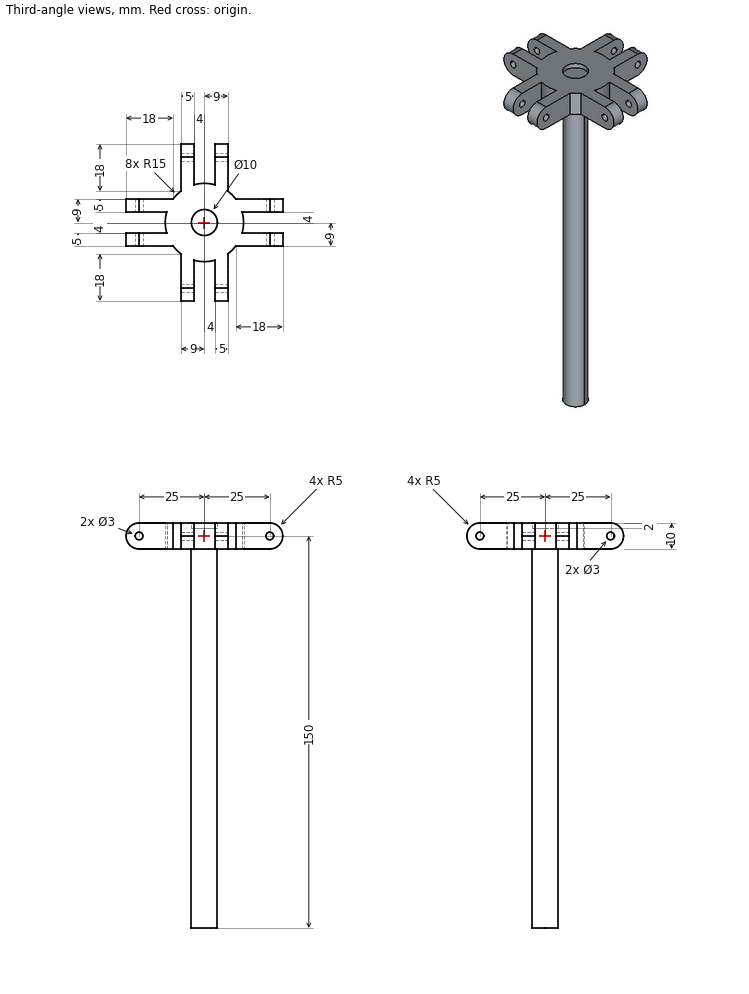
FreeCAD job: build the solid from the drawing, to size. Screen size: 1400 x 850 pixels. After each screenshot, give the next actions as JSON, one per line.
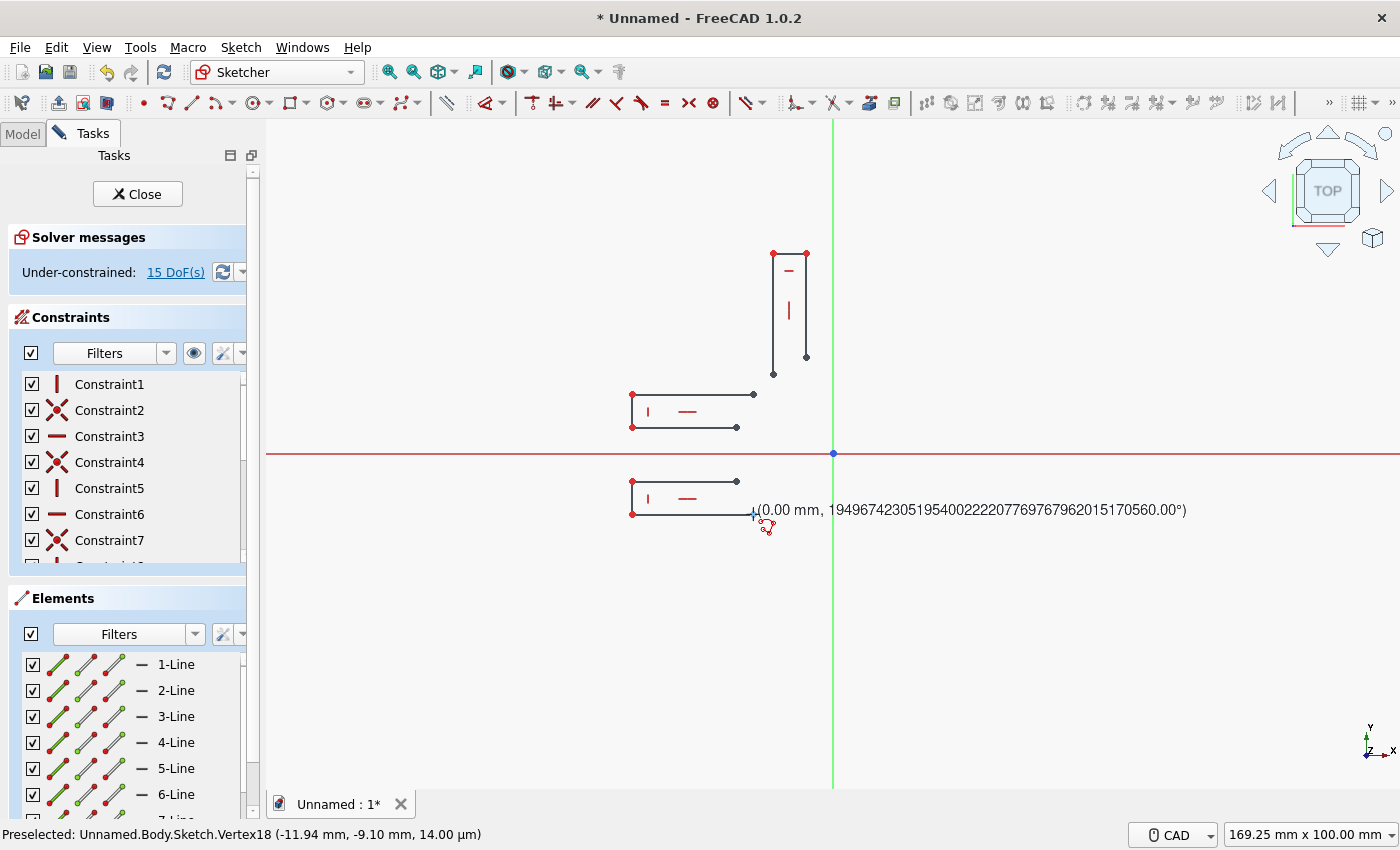
{"action": "left_click", "coordinate": [773, 534]}
{"action": "left_click", "coordinate": [773, 655]}
{"action": "left_click", "coordinate": [806, 655]}
{"action": "left_click", "coordinate": [806, 551]}
{"action": "right_click", "coordinate": [806, 551]}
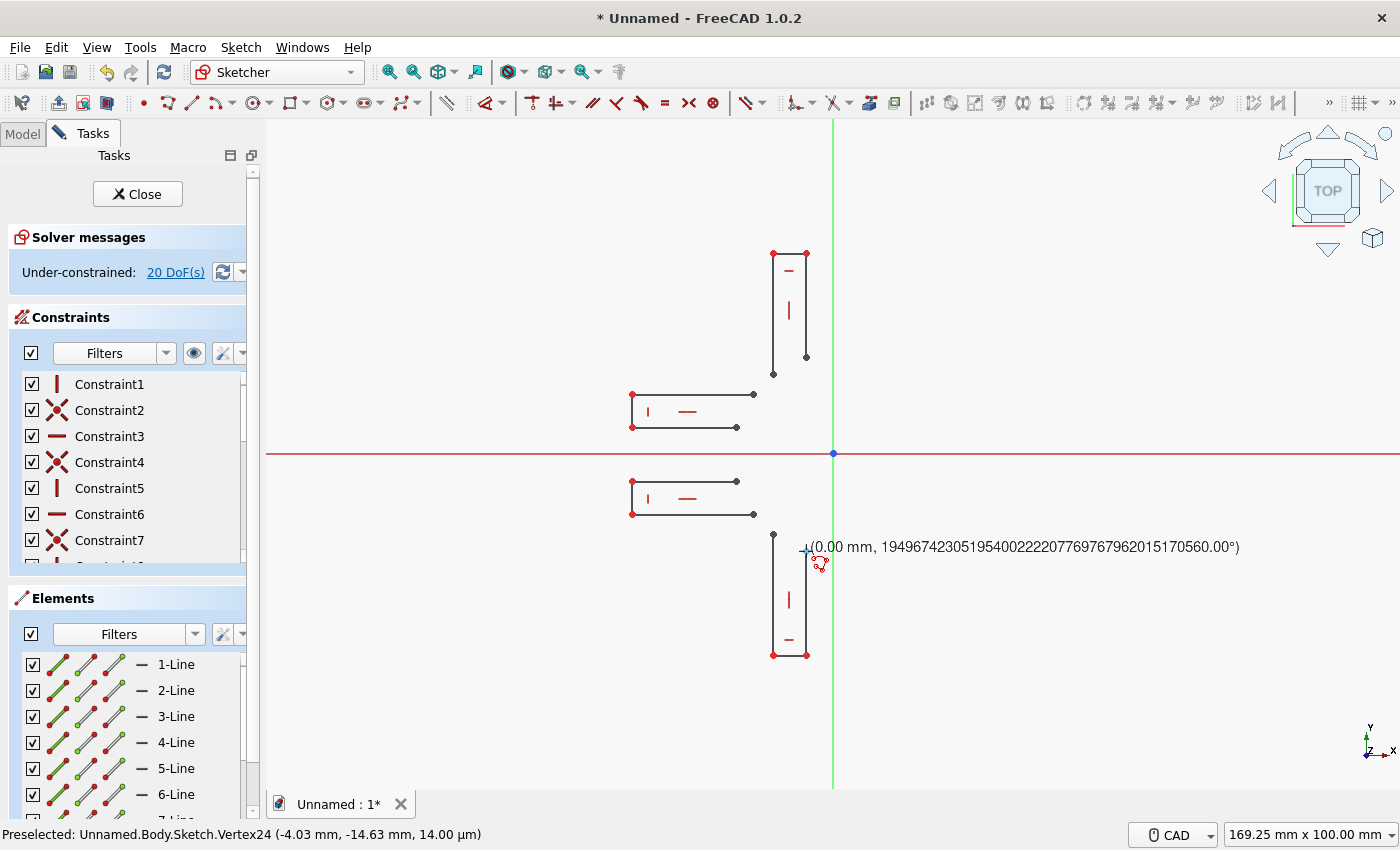
{"action": "left_click", "coordinate": [860, 551]}
{"action": "left_click", "coordinate": [860, 655]}
{"action": "left_click", "coordinate": [893, 655]}
{"action": "left_click", "coordinate": [893, 534]}
{"action": "right_click", "coordinate": [893, 534]}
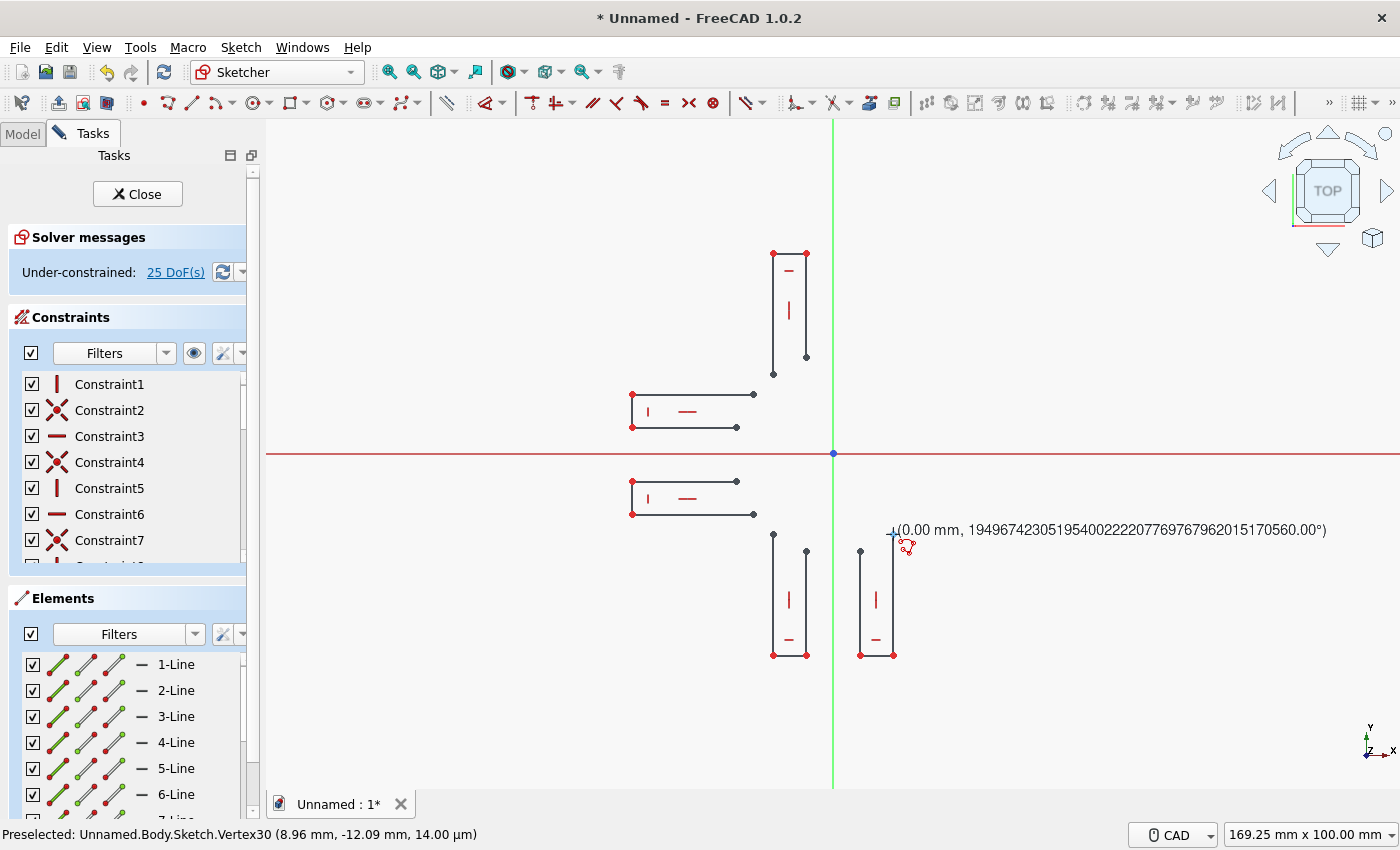
{"action": "left_click", "coordinate": [913, 514]}
{"action": "left_click", "coordinate": [1034, 514]}
{"action": "left_click", "coordinate": [1034, 481]}
{"action": "left_click", "coordinate": [930, 481]}
{"action": "right_click", "coordinate": [930, 481]}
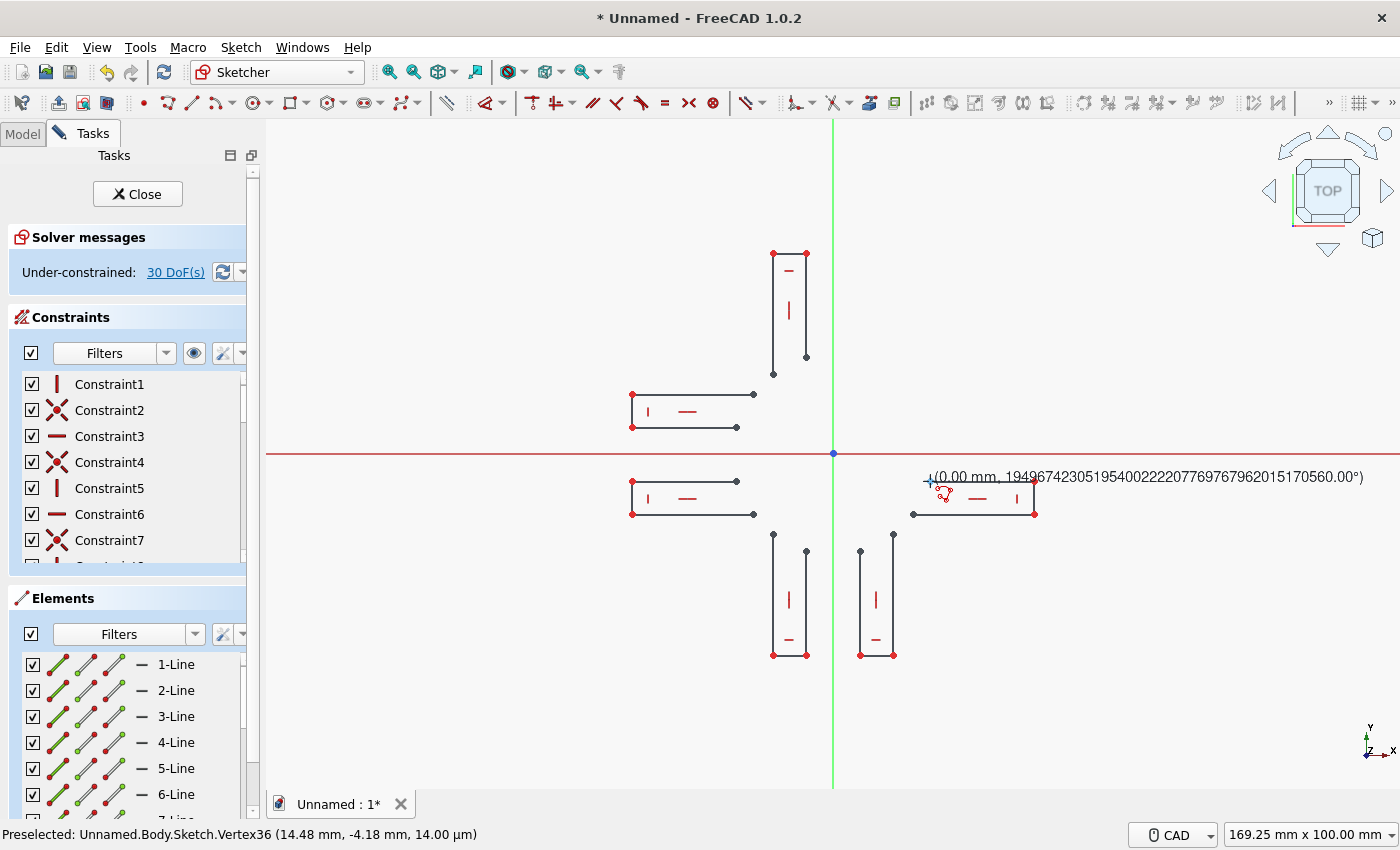
{"action": "left_click", "coordinate": [930, 427]}
{"action": "left_click", "coordinate": [1034, 427]}
{"action": "left_click", "coordinate": [1034, 394]}
{"action": "left_click", "coordinate": [913, 394]}
{"action": "right_click", "coordinate": [913, 394]}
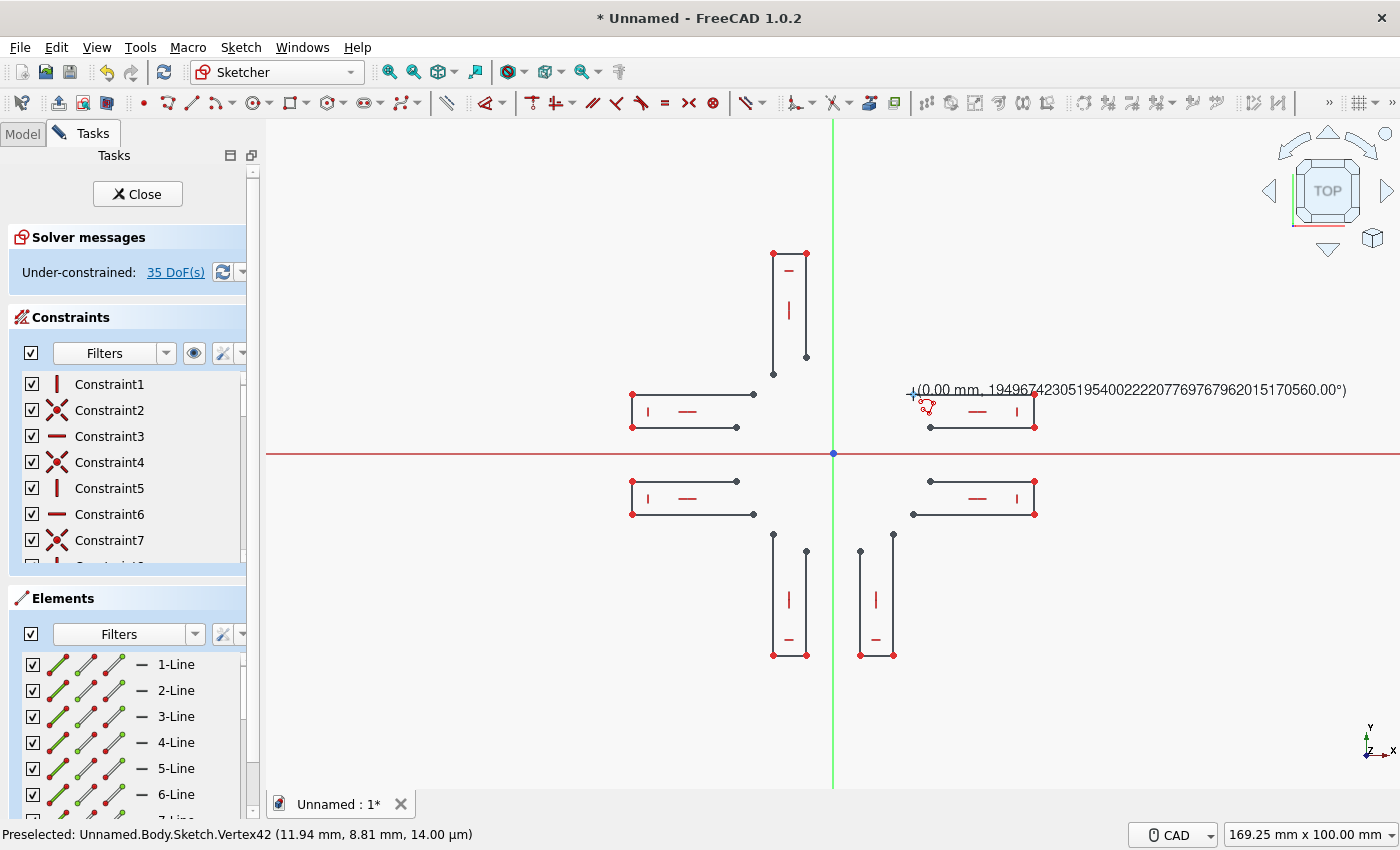
{"action": "left_click", "coordinate": [893, 374]}
{"action": "left_click", "coordinate": [893, 253]}
{"action": "left_click", "coordinate": [860, 253]}
{"action": "left_click", "coordinate": [860, 357]}
{"action": "right_click", "coordinate": [860, 357]}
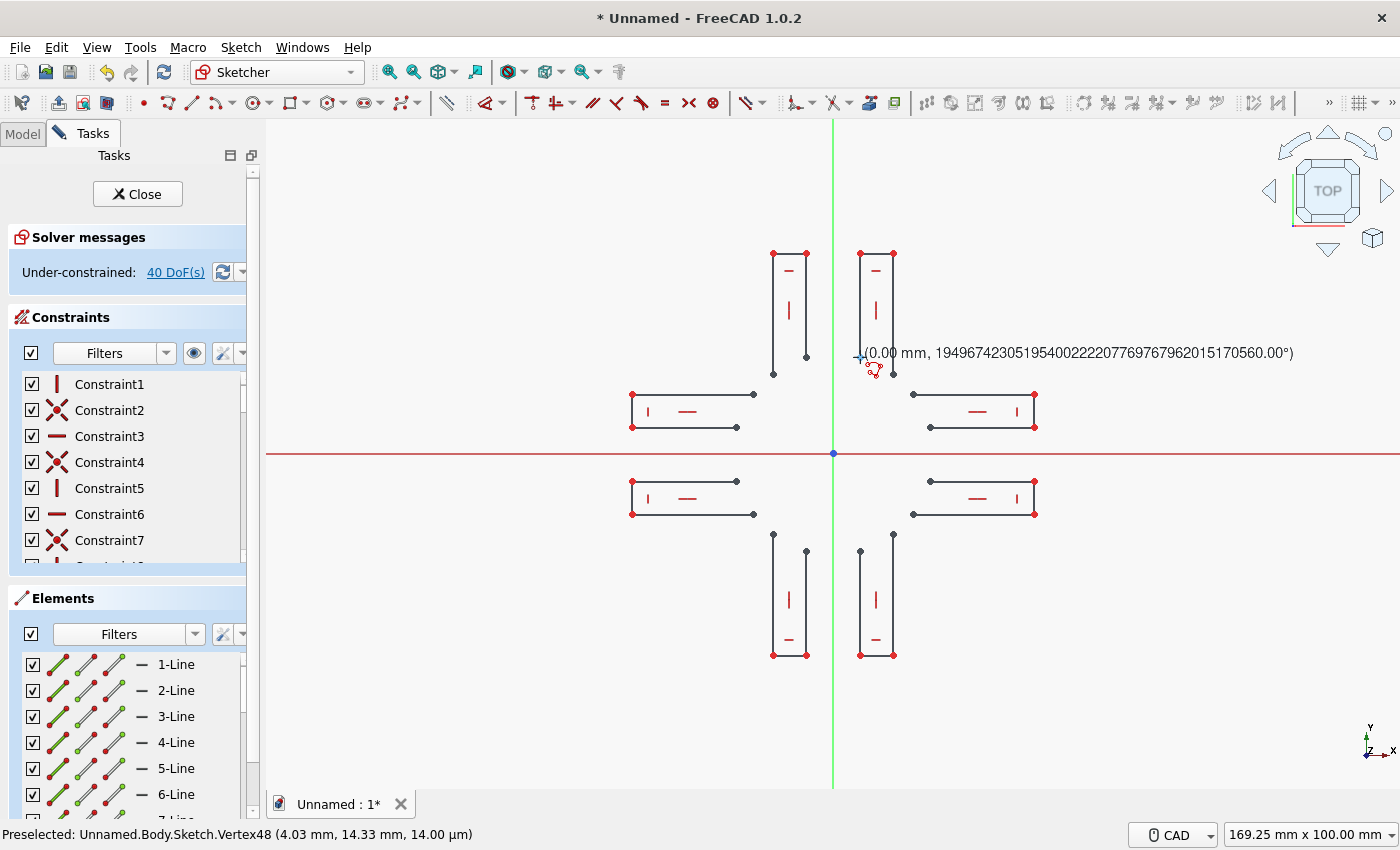
{"action": "key", "text": "g 3 a"}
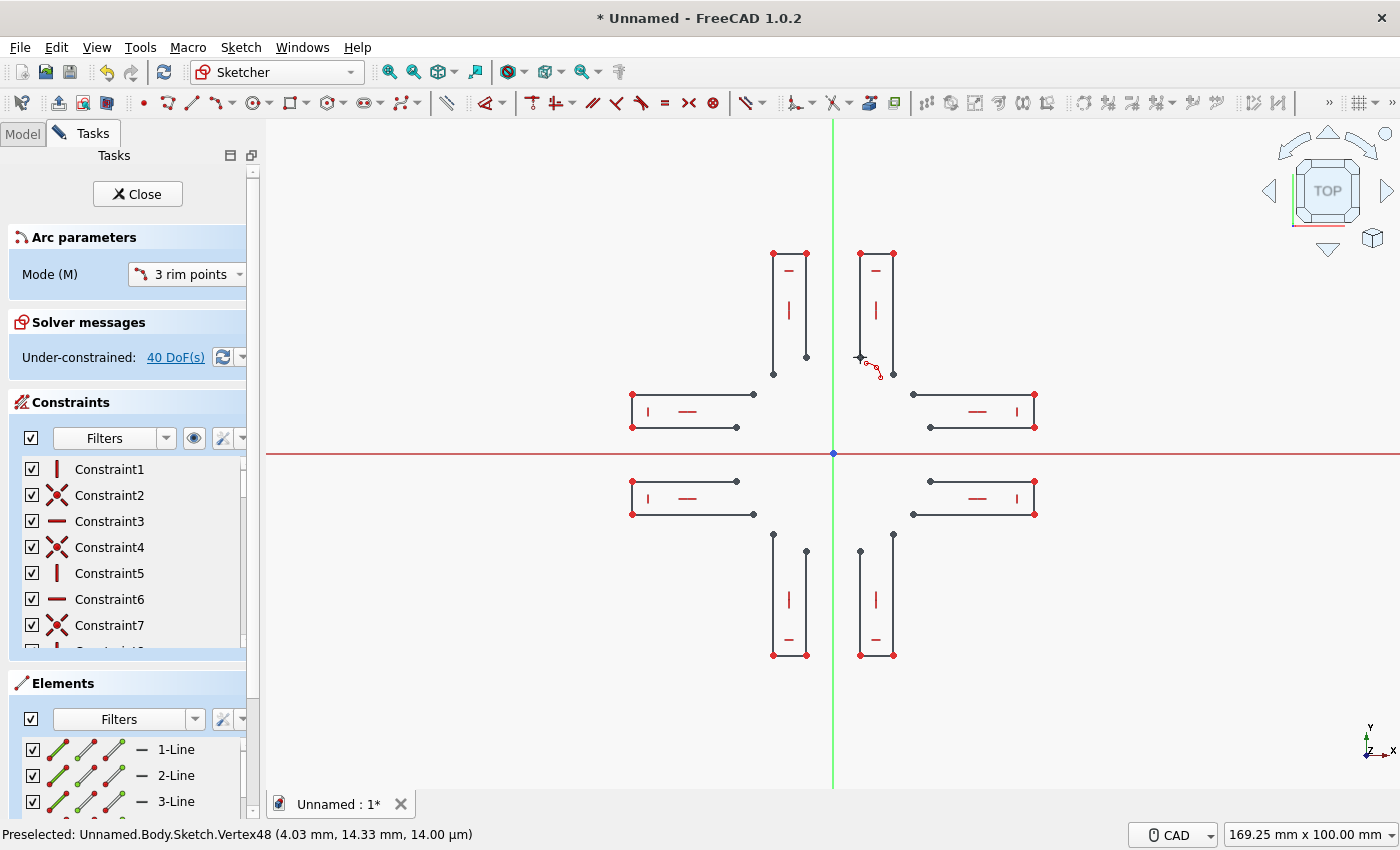
{"action": "left_click", "coordinate": [773, 375]}
{"action": "left_click", "coordinate": [753, 395]}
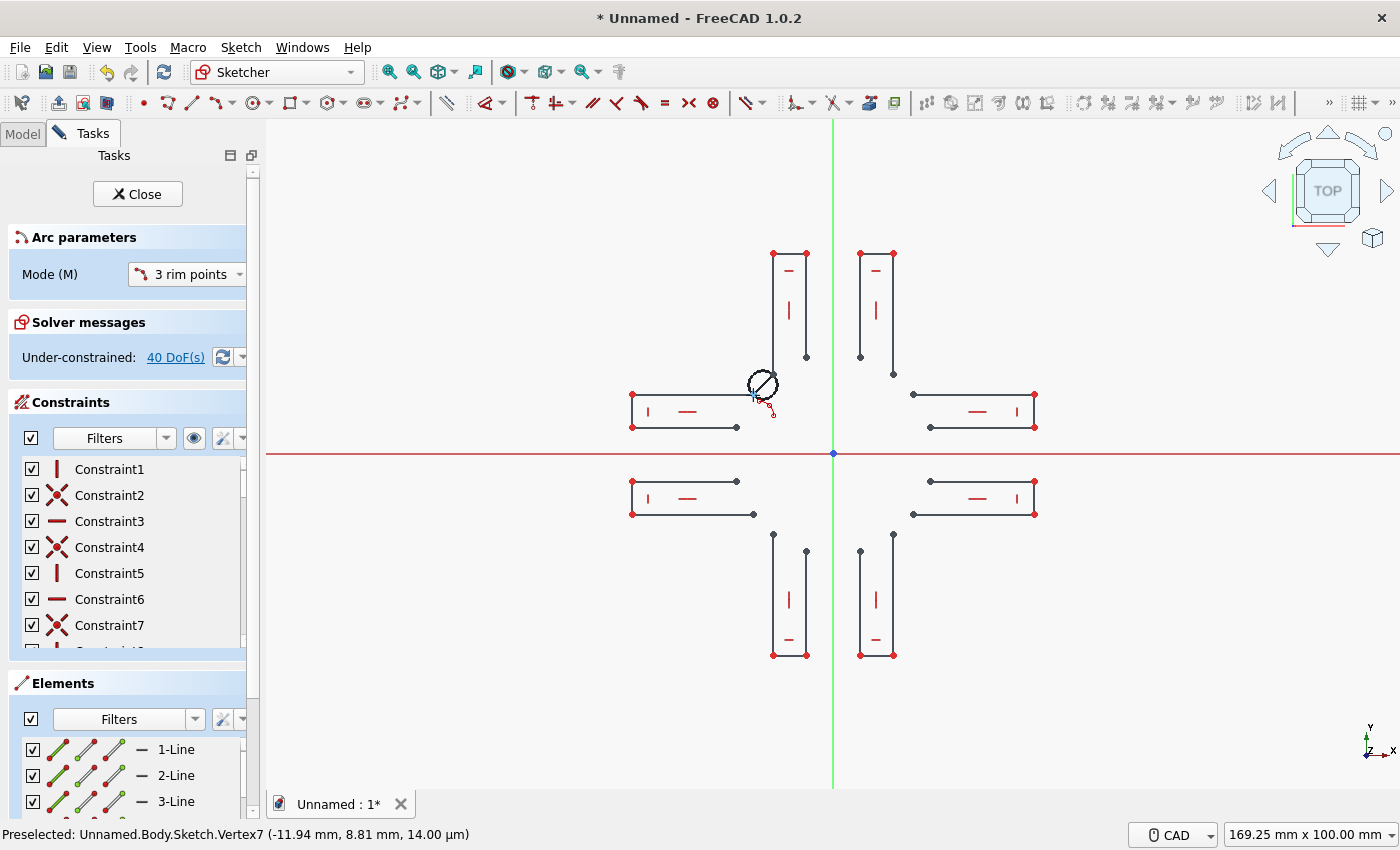
{"action": "scroll", "coordinate": [762, 383], "scroll_direction": "up", "scroll_amount": 14}